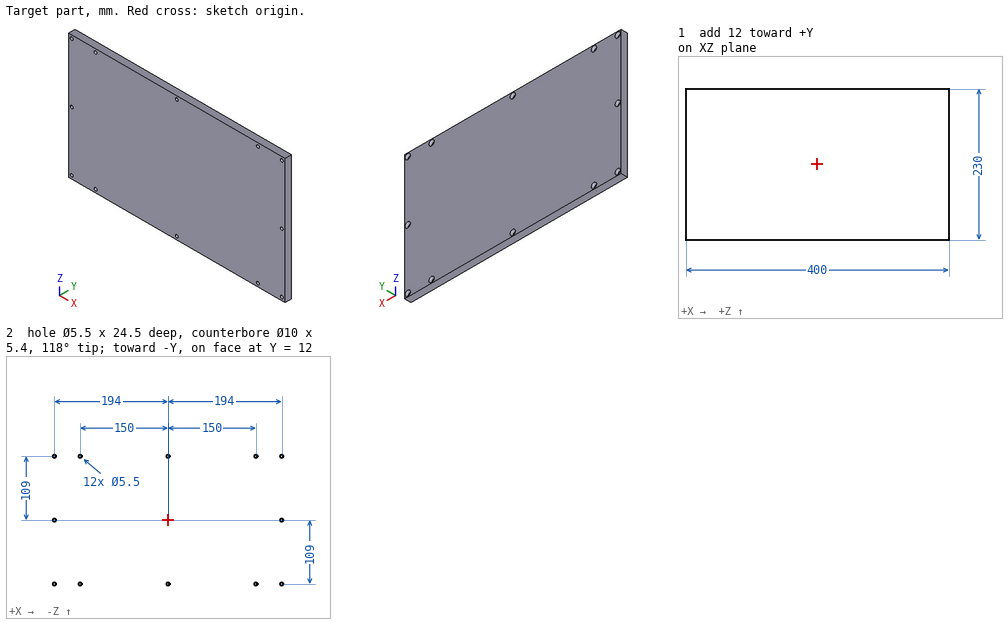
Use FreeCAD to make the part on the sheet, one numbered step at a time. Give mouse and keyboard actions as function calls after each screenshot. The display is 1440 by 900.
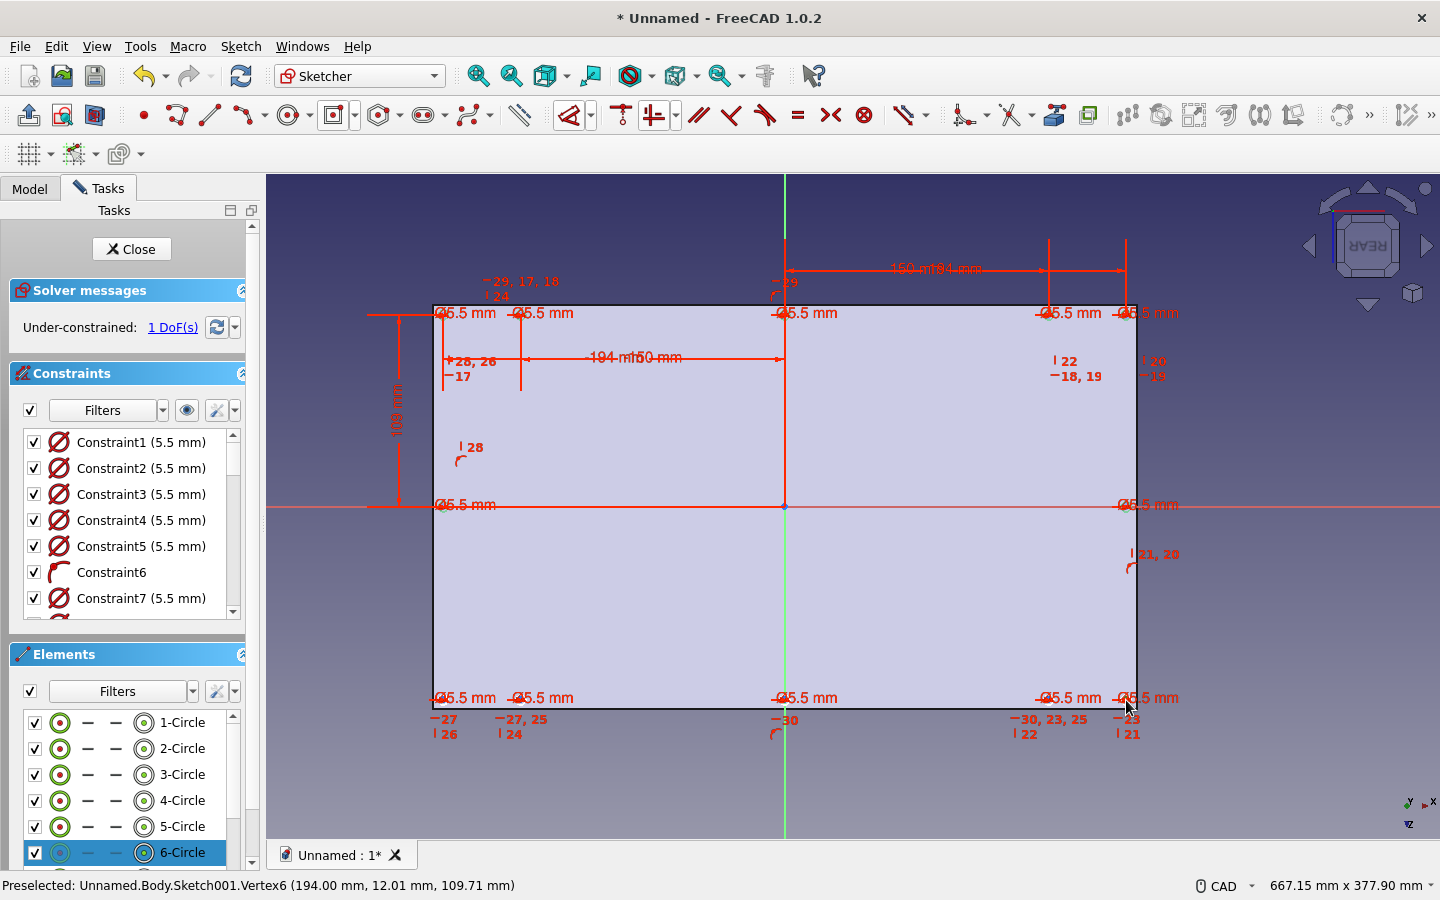
click(590, 116)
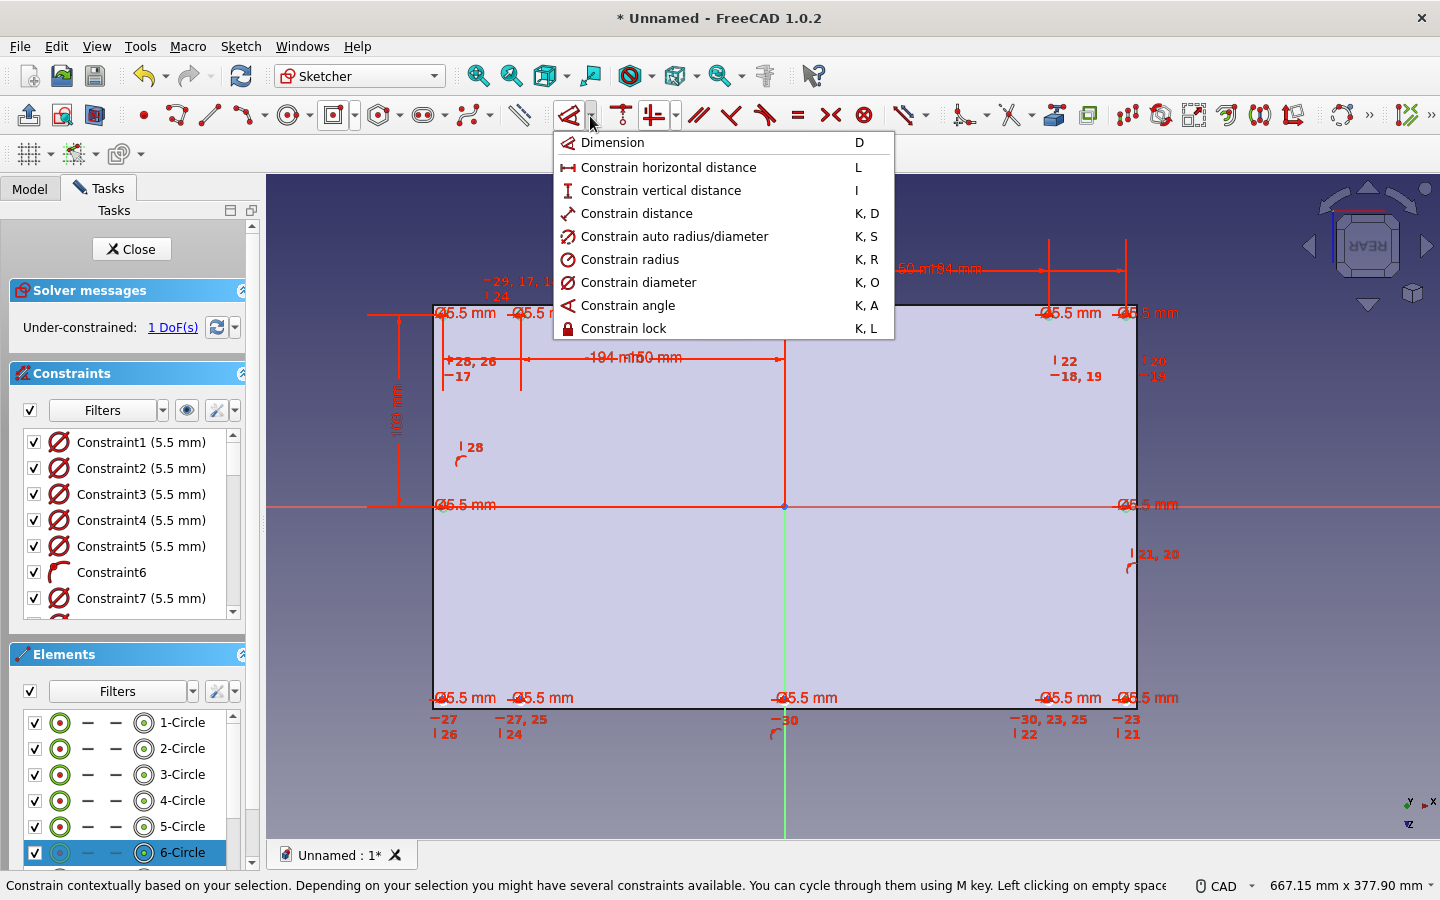
click(724, 190)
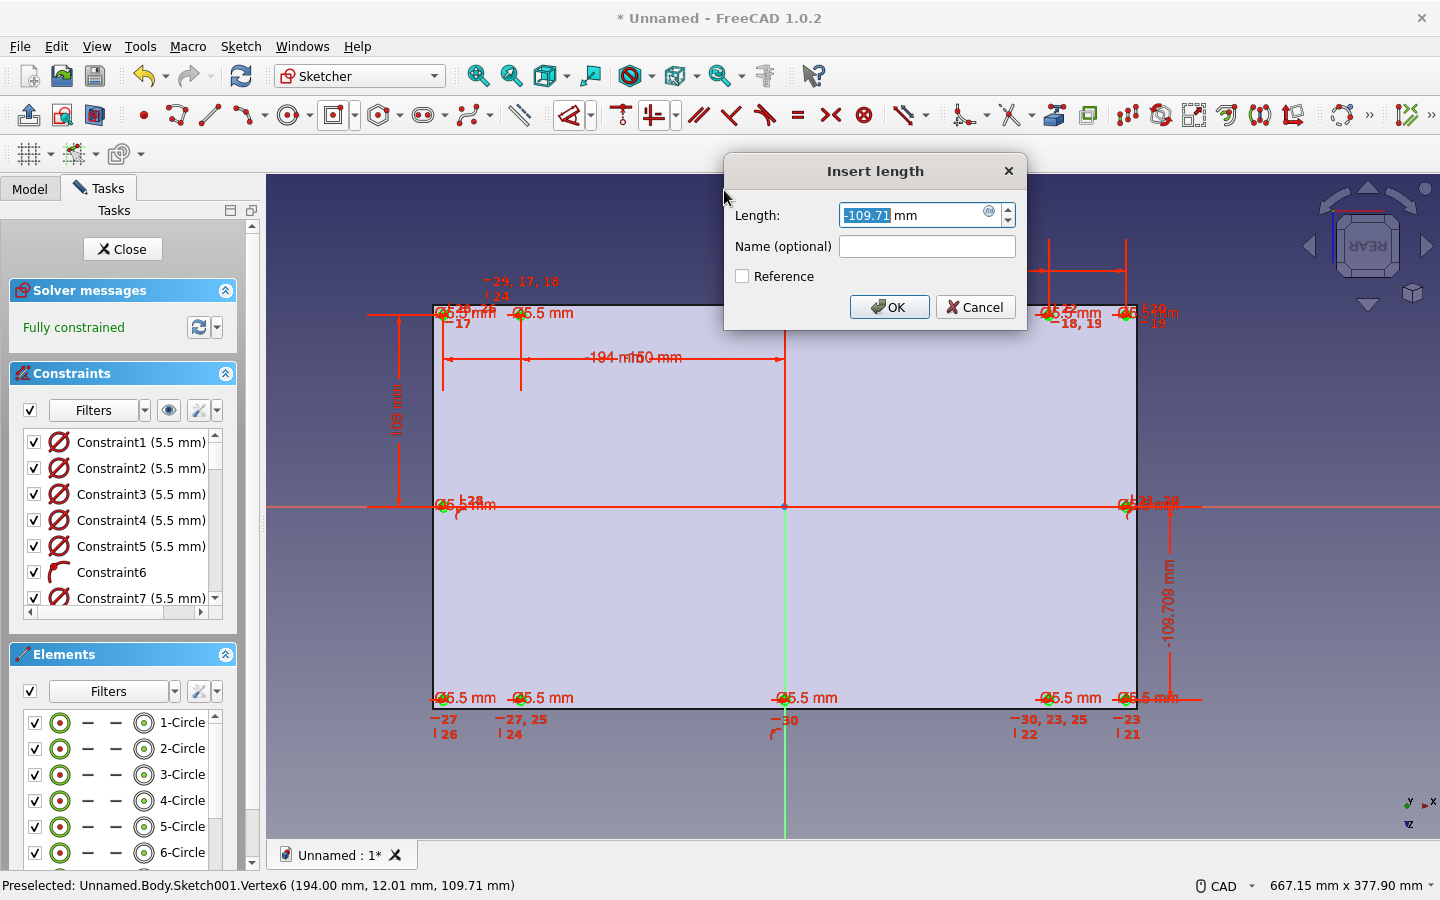
text(-109)
key(Return)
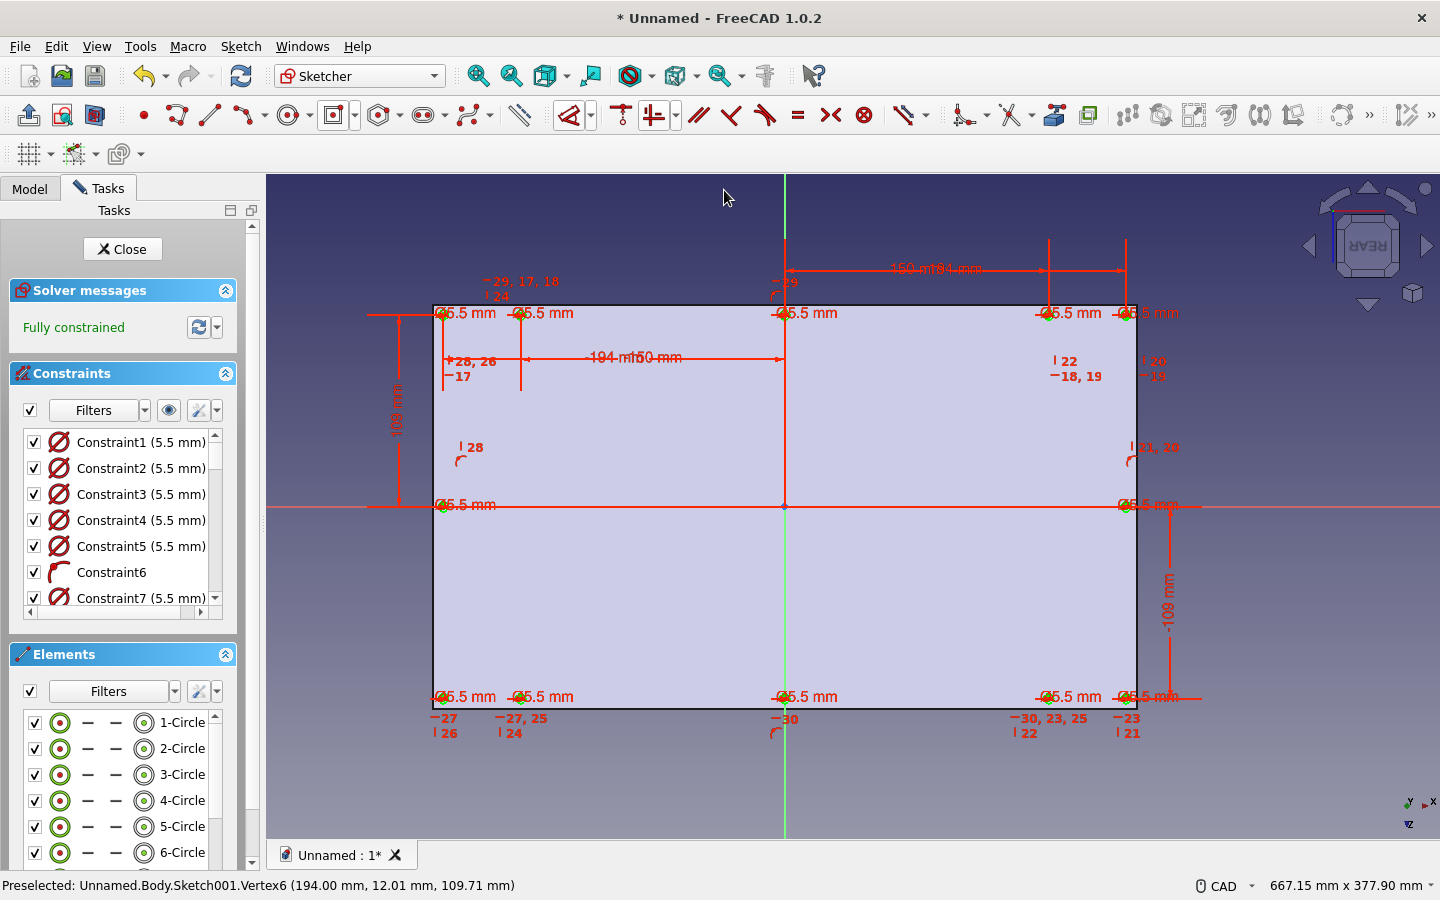
click(123, 249)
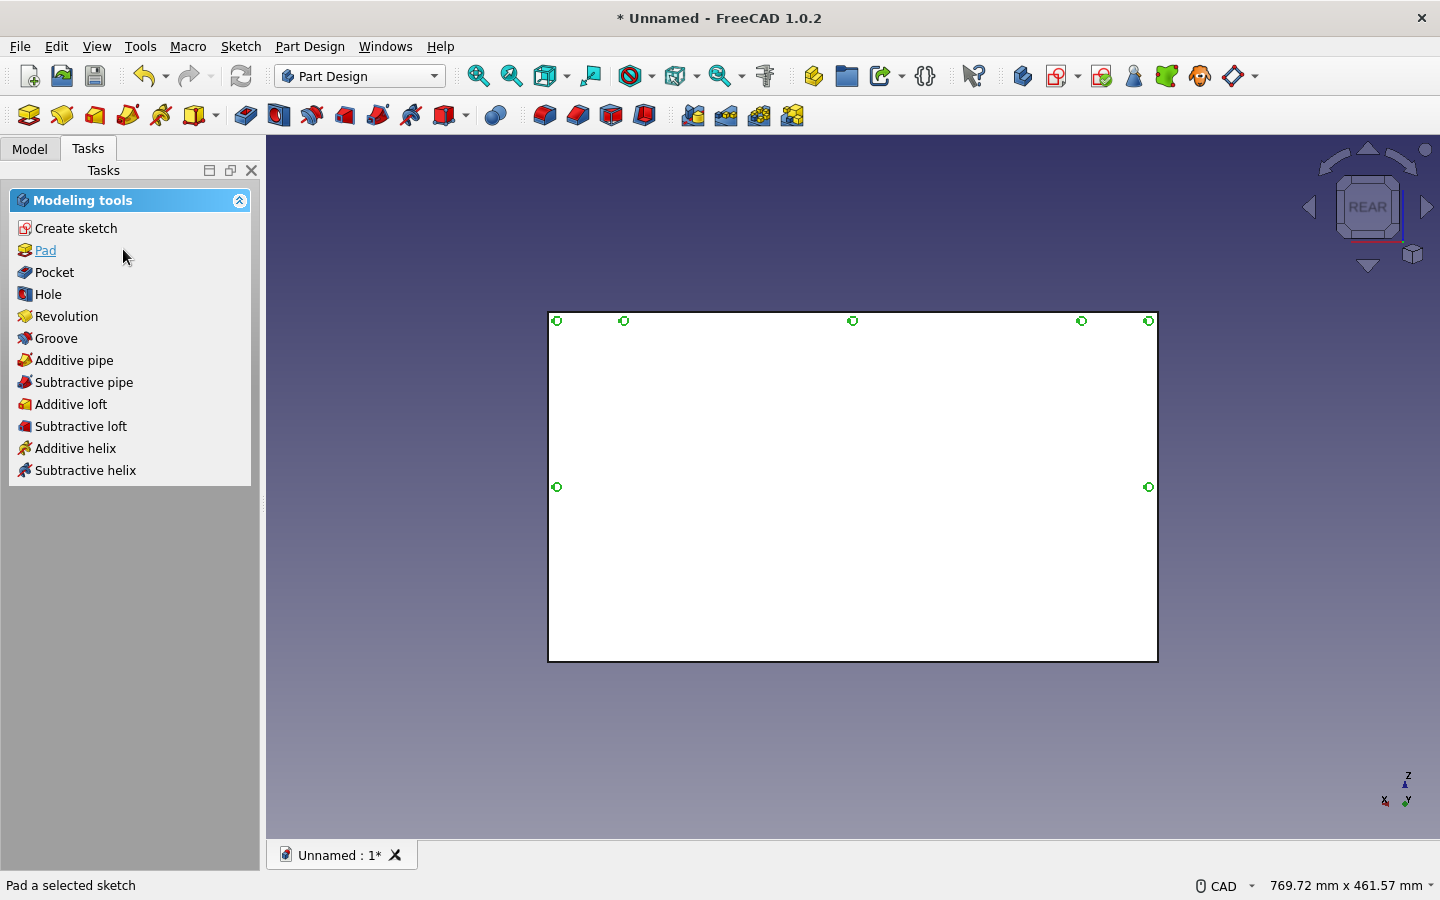
click(279, 116)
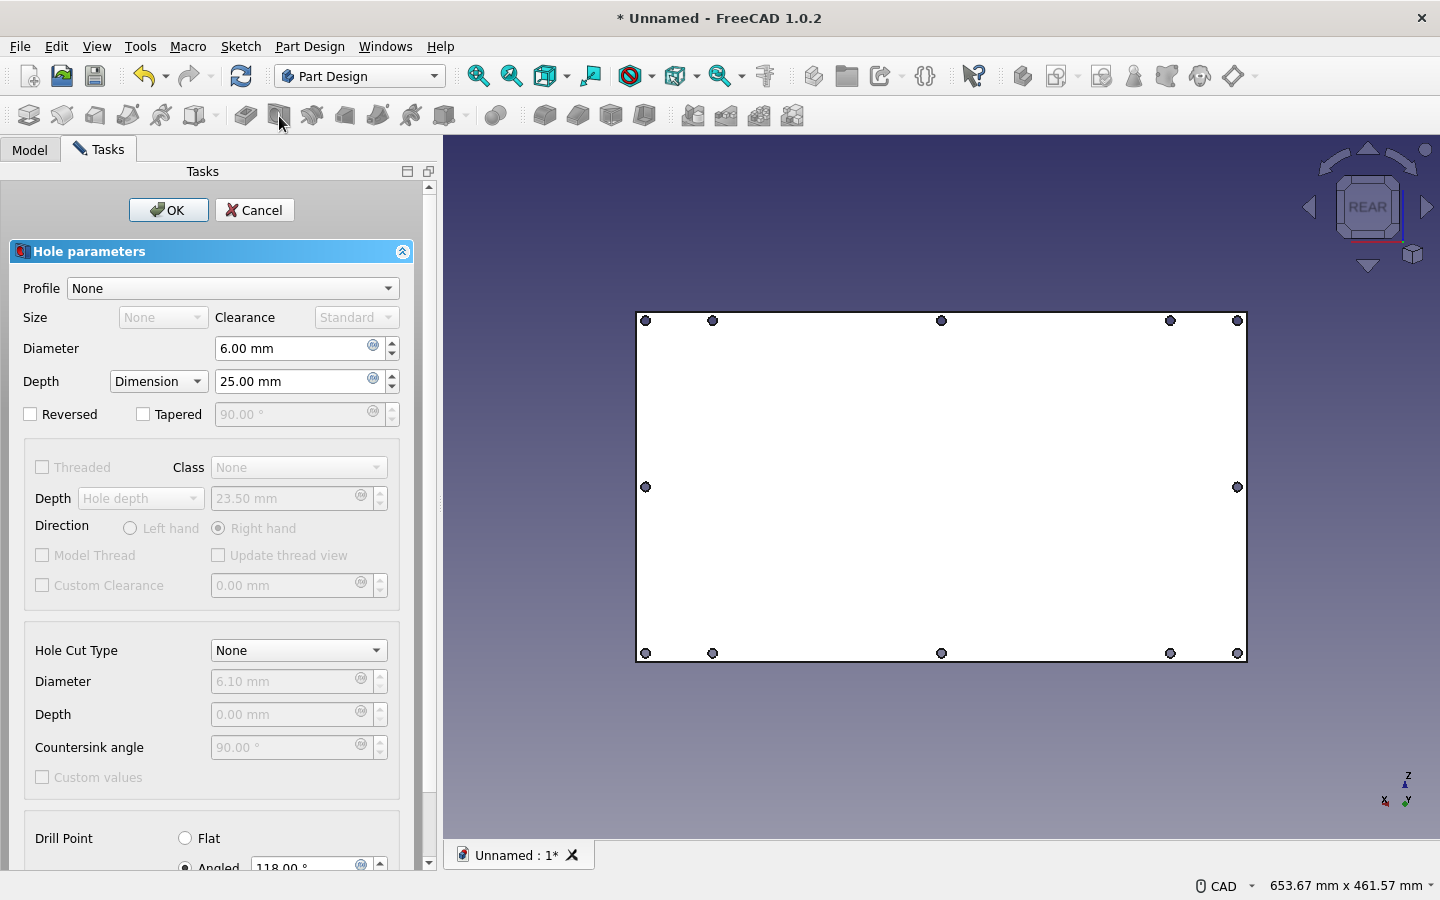
triple_click(300, 348)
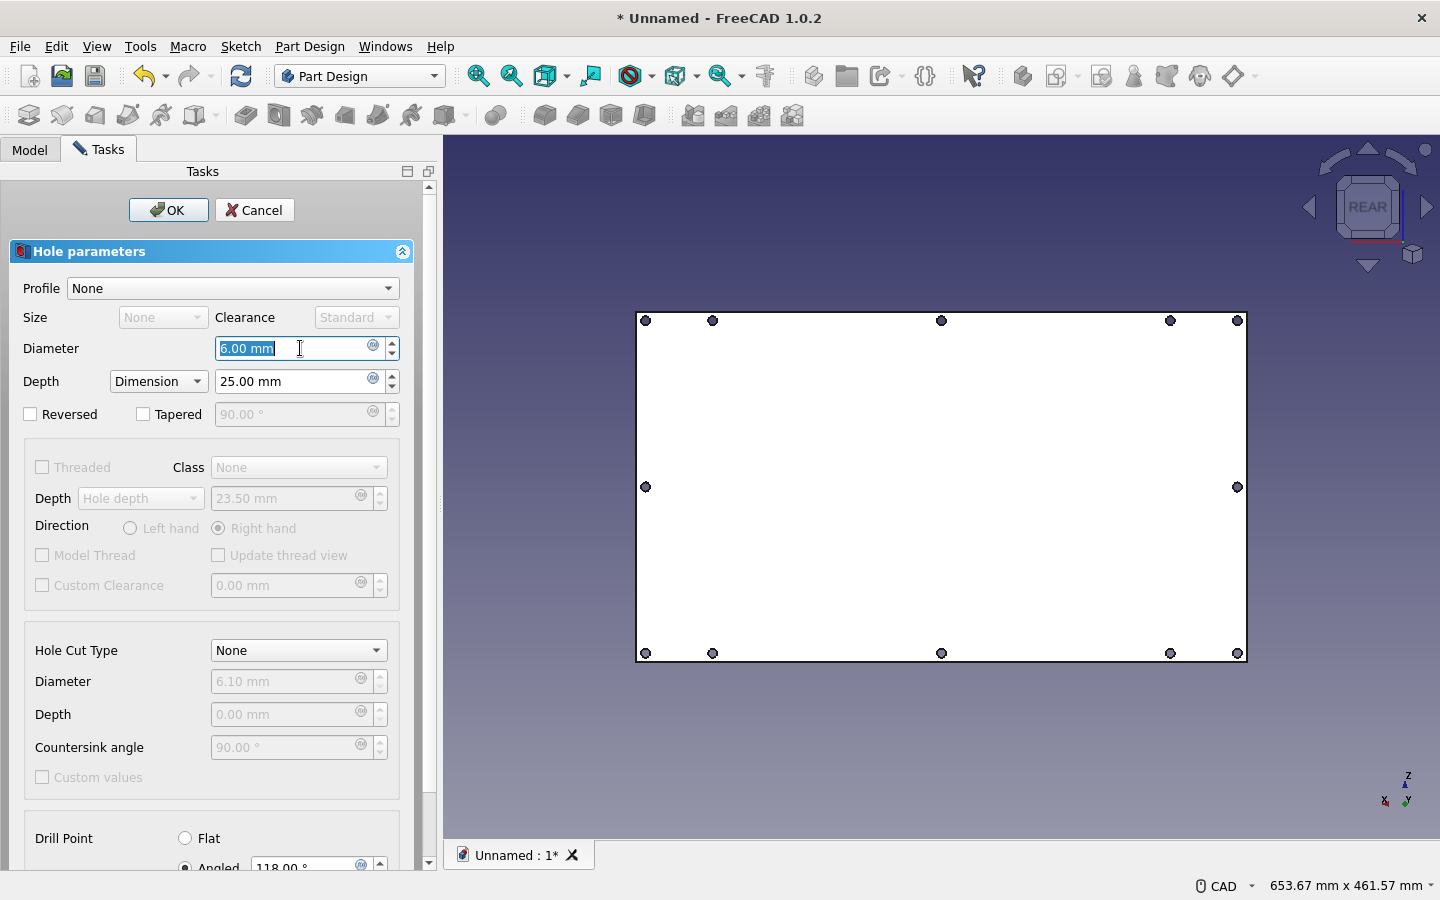
text(5.5)
key(Tab)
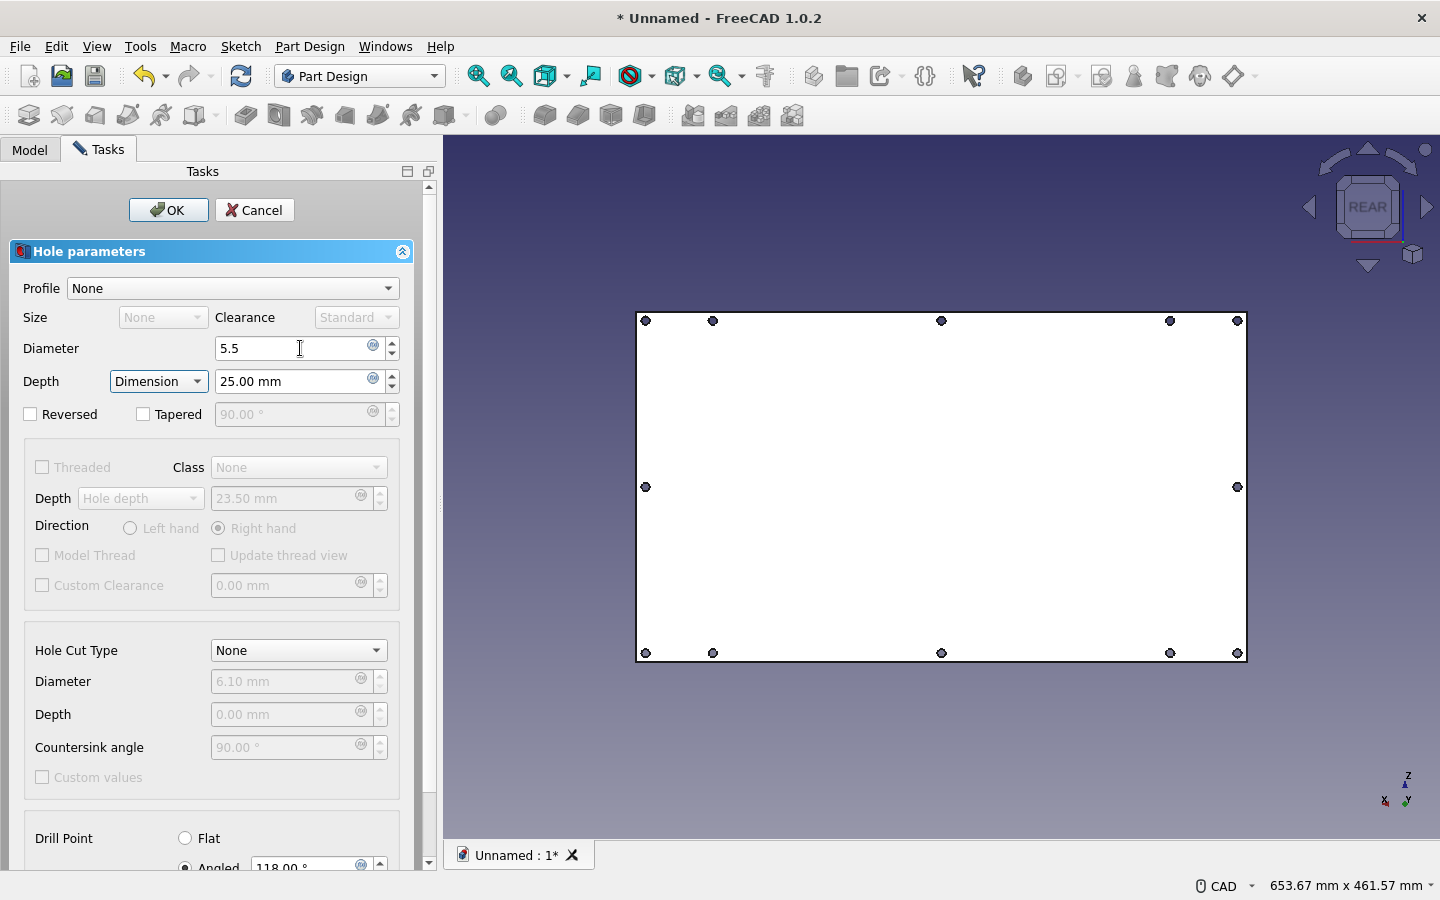
triple_click(300, 382)